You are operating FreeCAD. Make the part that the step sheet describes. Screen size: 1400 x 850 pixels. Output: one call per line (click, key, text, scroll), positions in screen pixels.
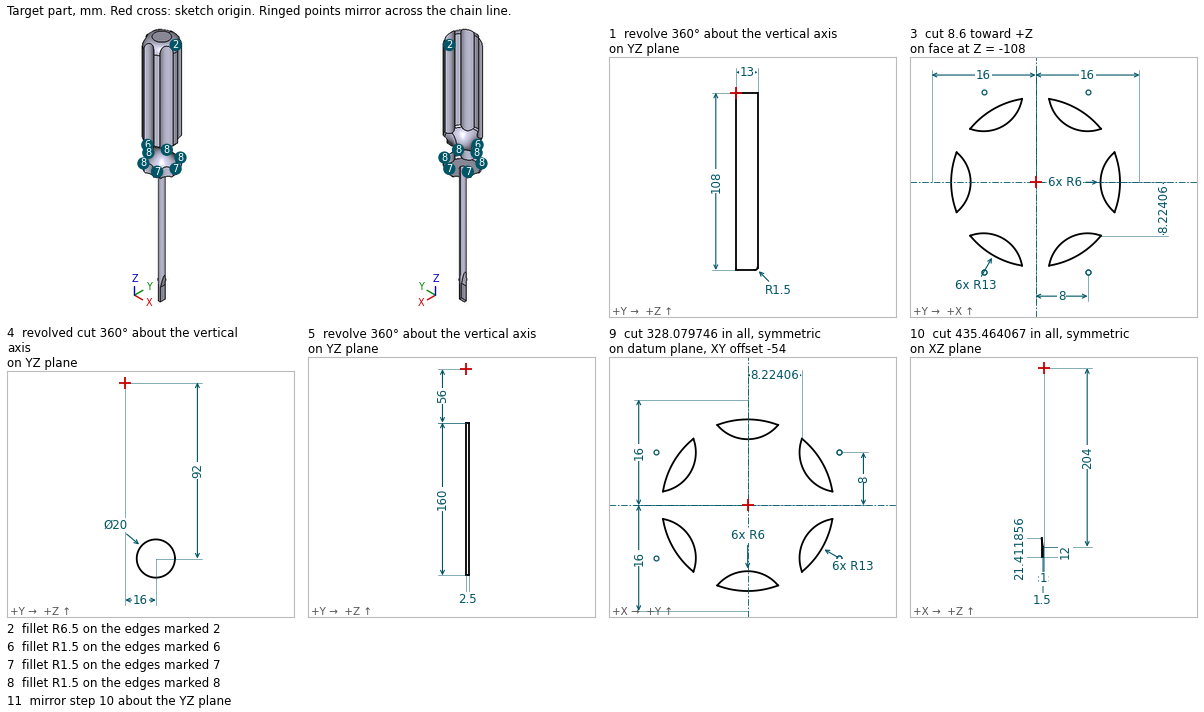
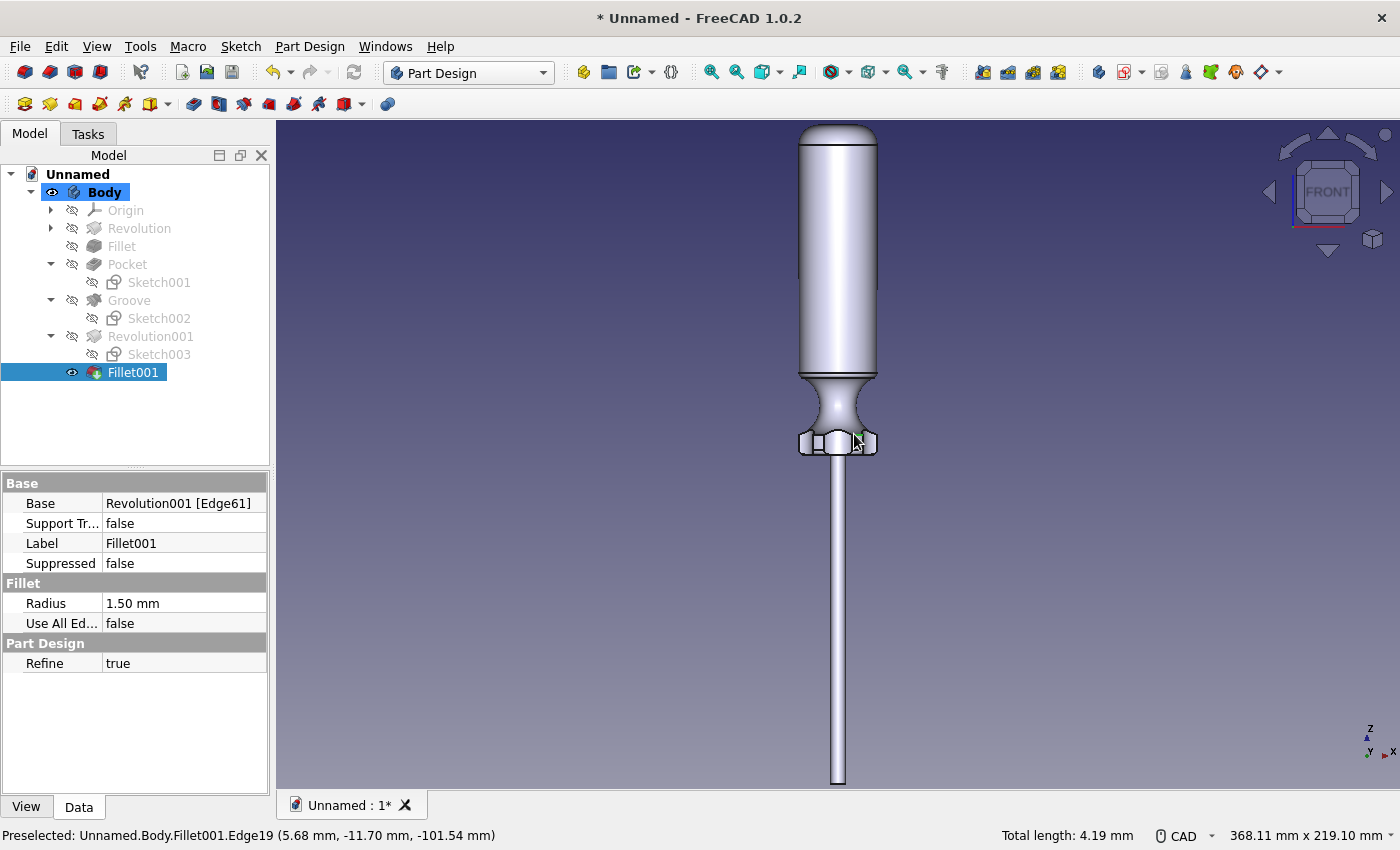
scroll(878, 434, up, 6)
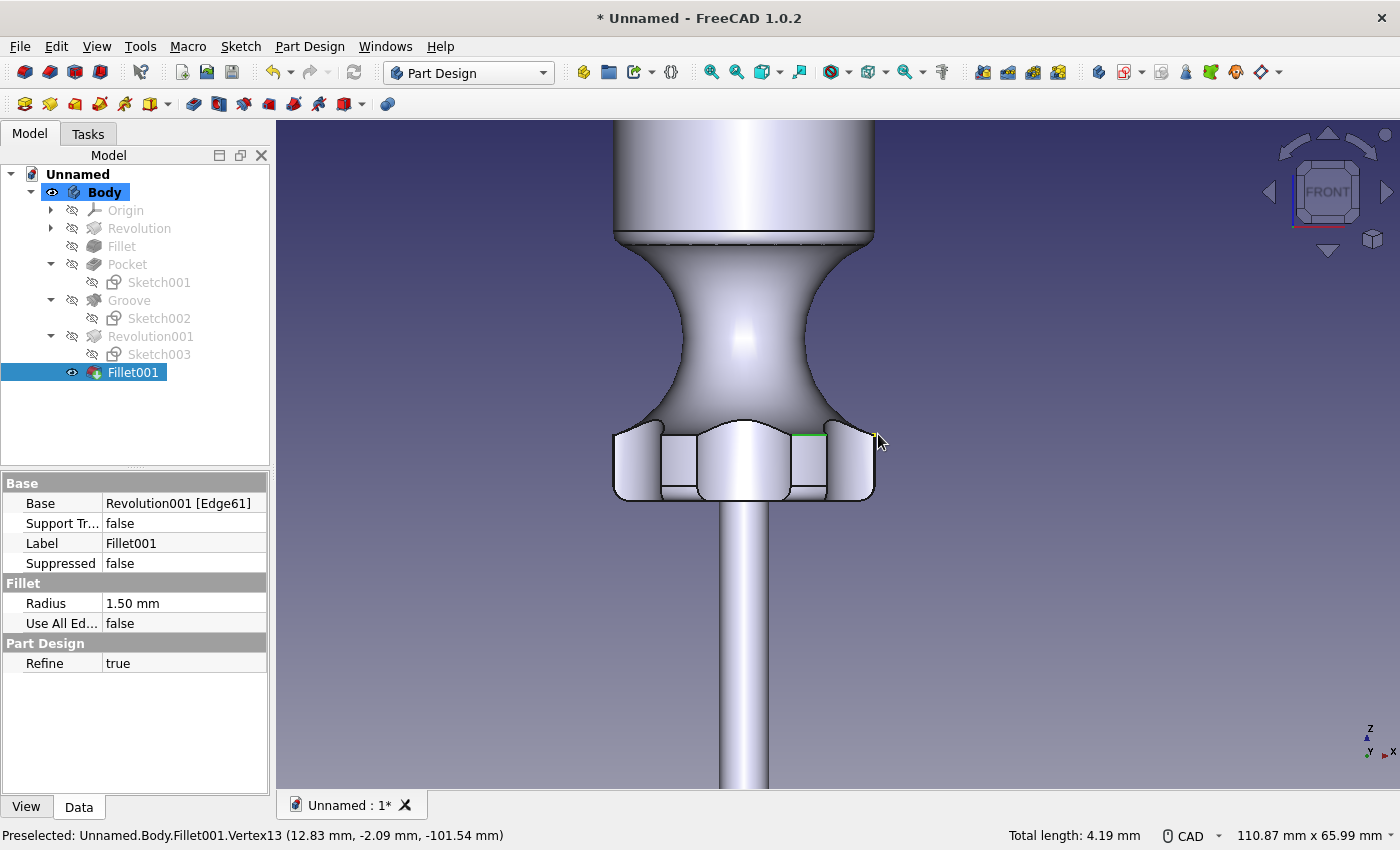
key(v)
key(f)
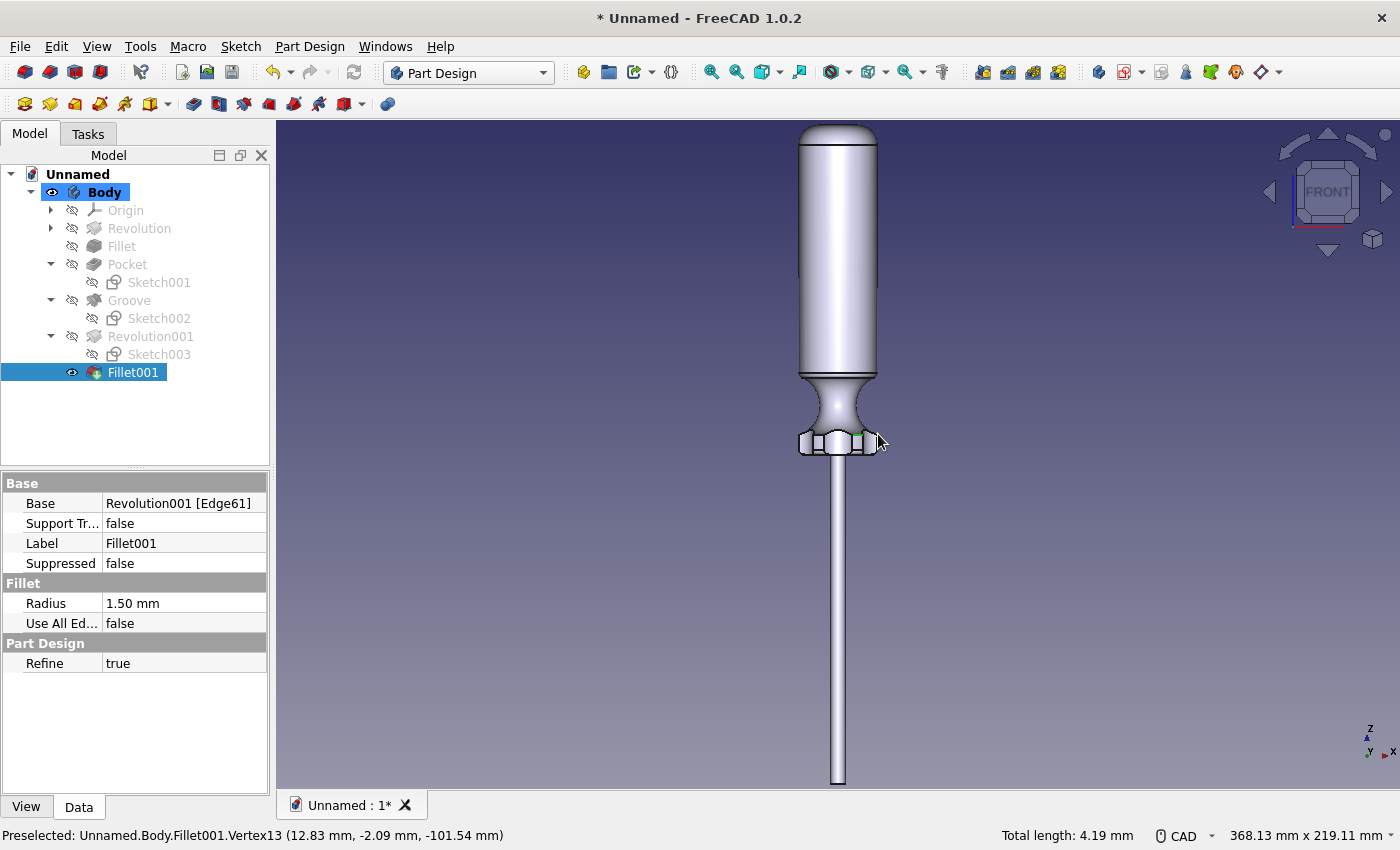
key(0)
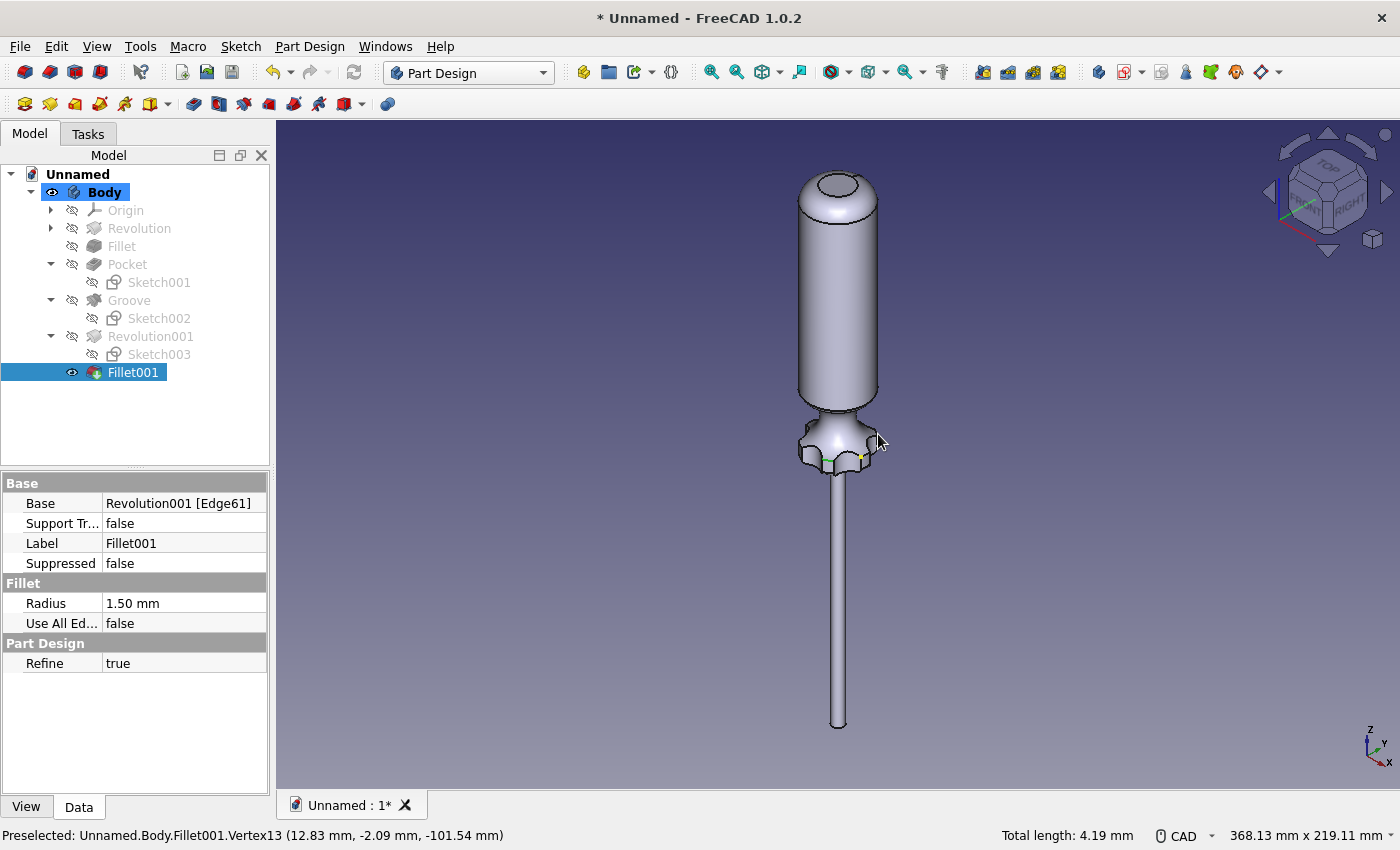
click(867, 453, ctrl)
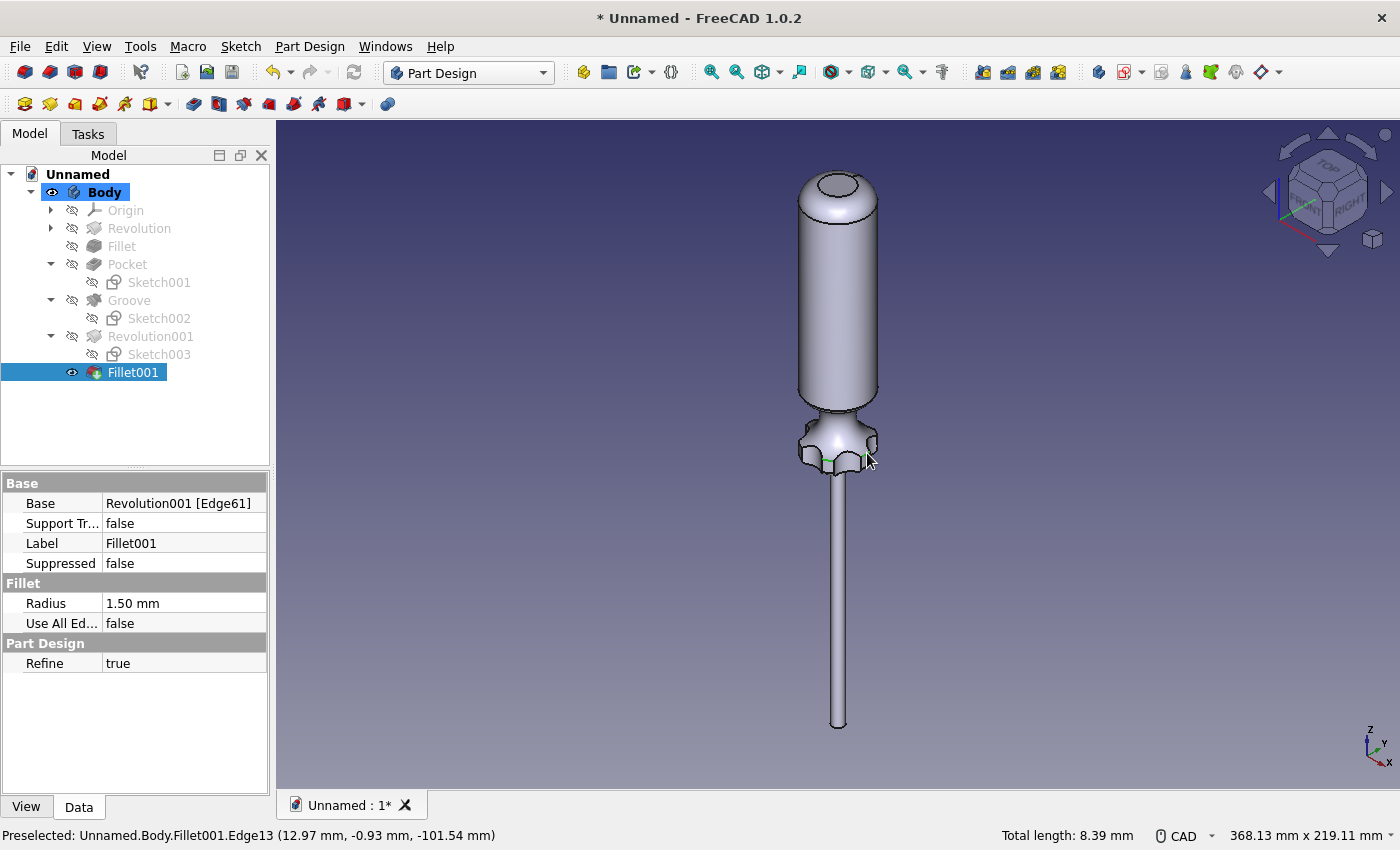
click(25, 72)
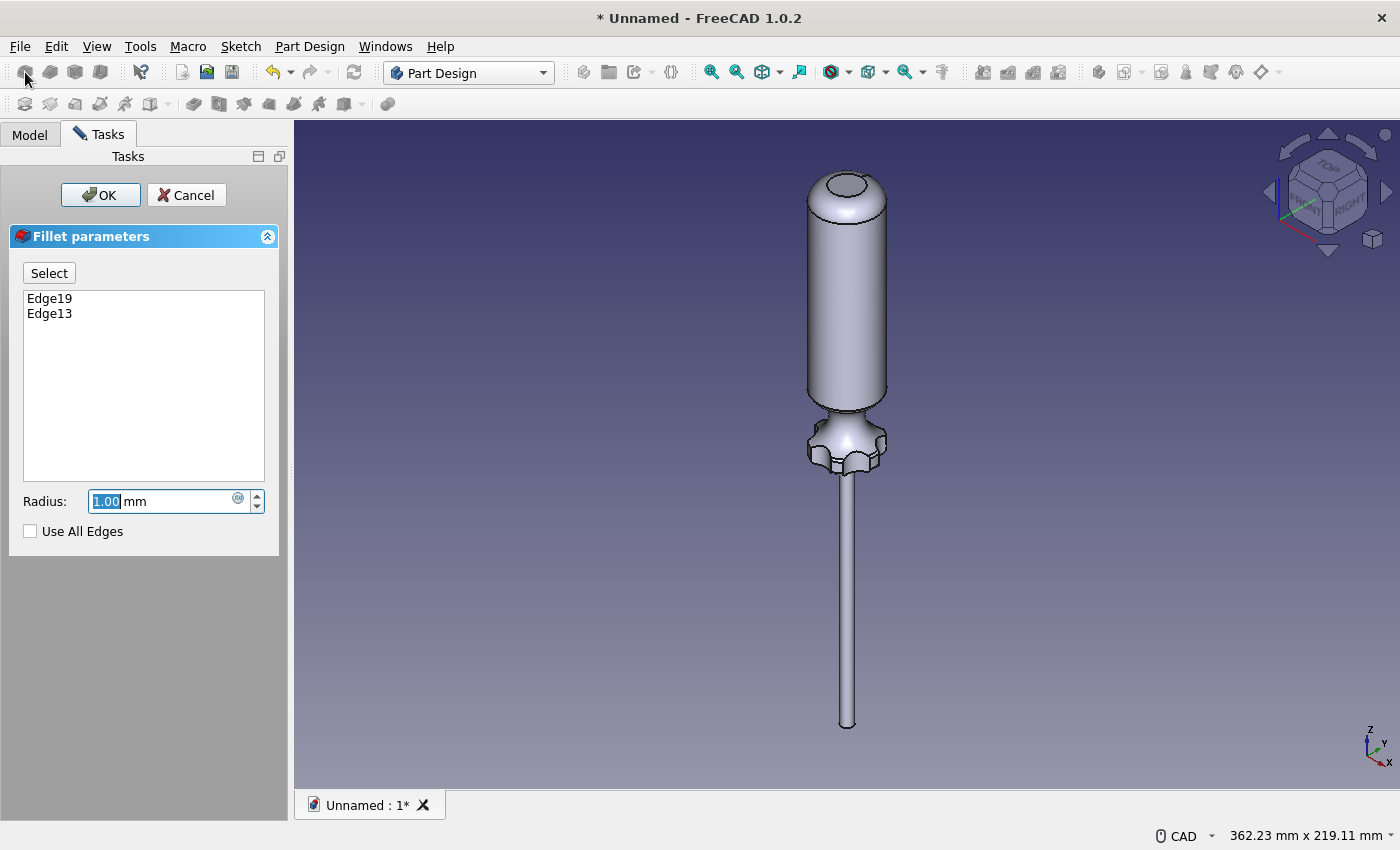
text(1.5)
key(Tab)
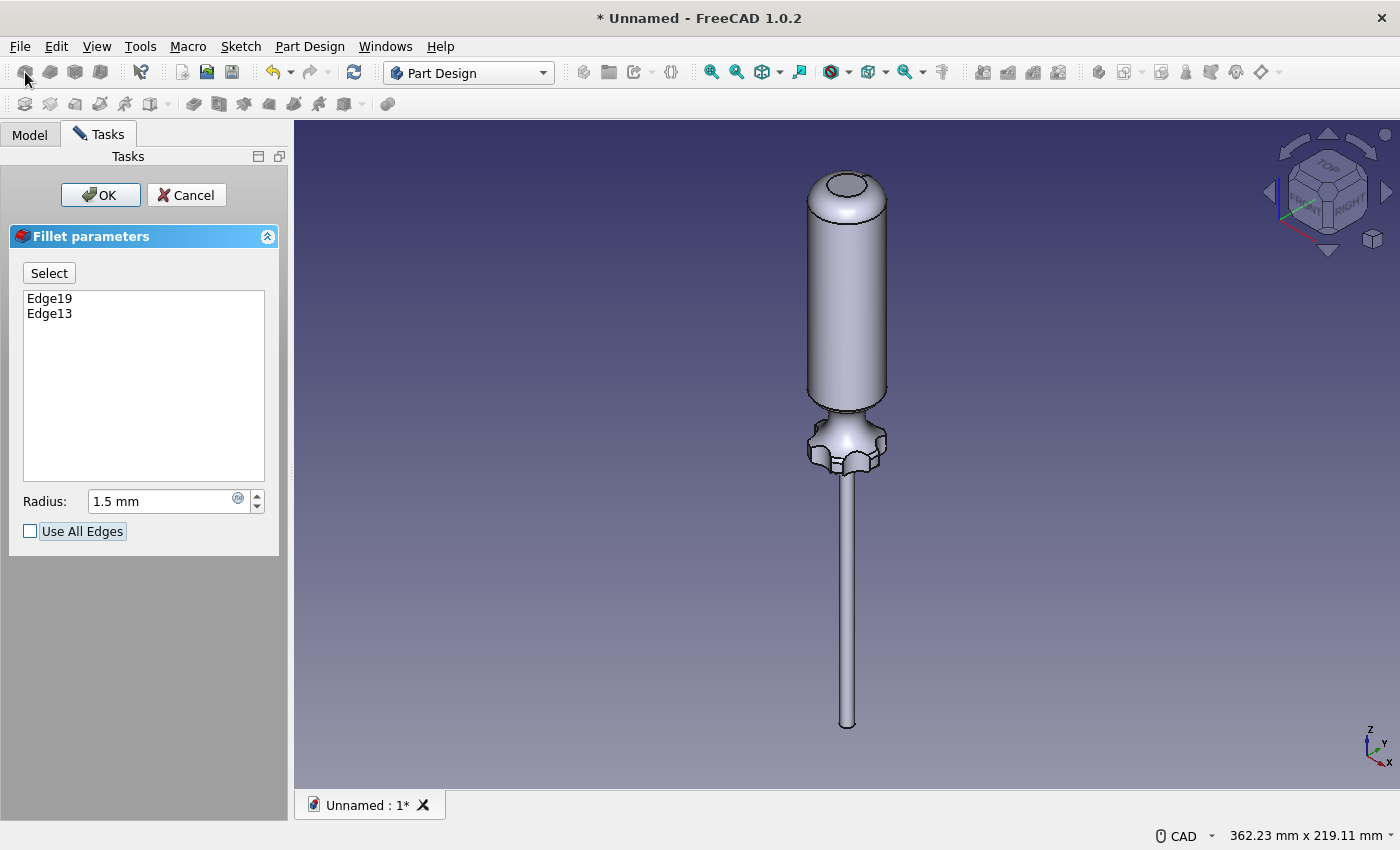
click(101, 195)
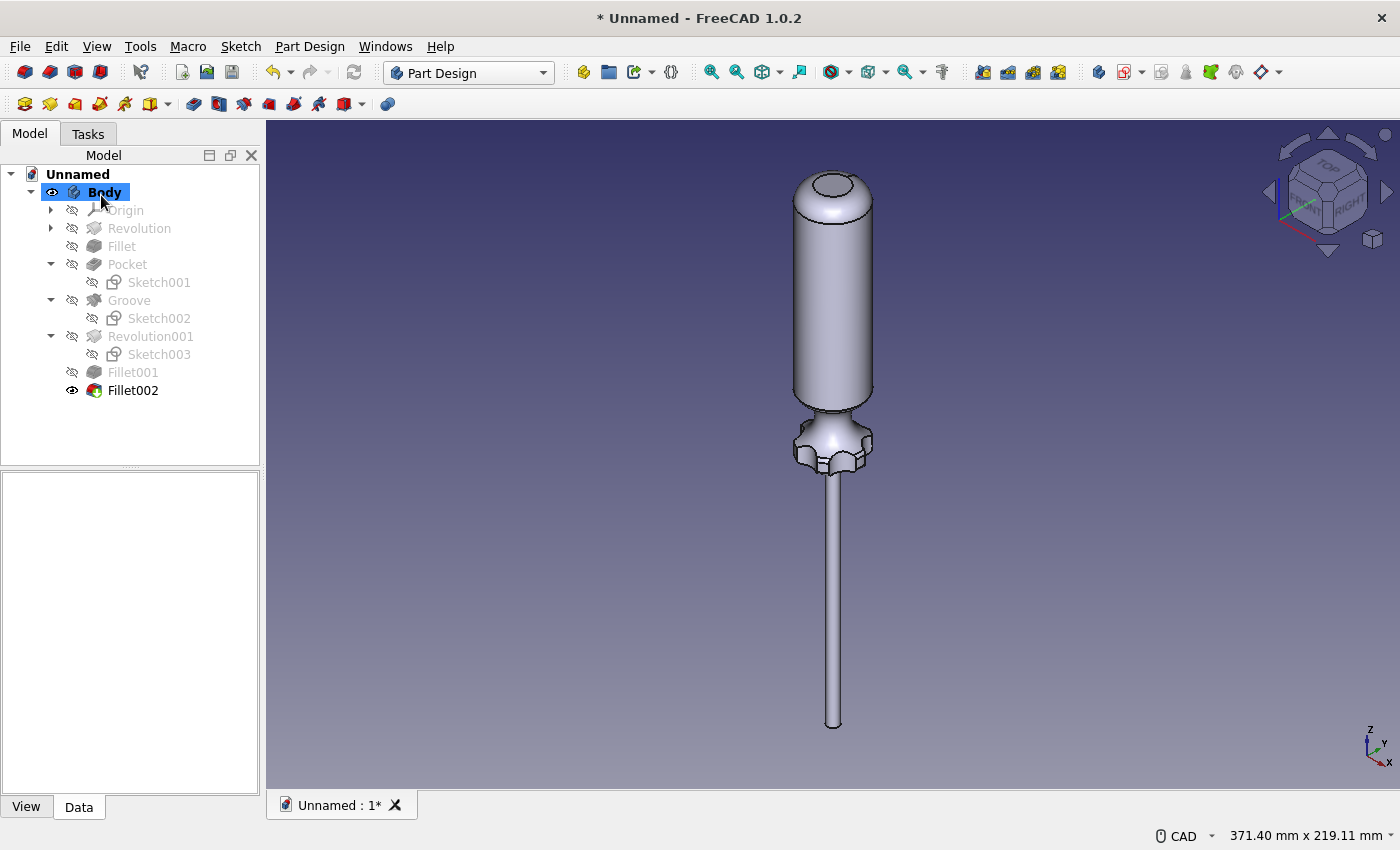
click(794, 441)